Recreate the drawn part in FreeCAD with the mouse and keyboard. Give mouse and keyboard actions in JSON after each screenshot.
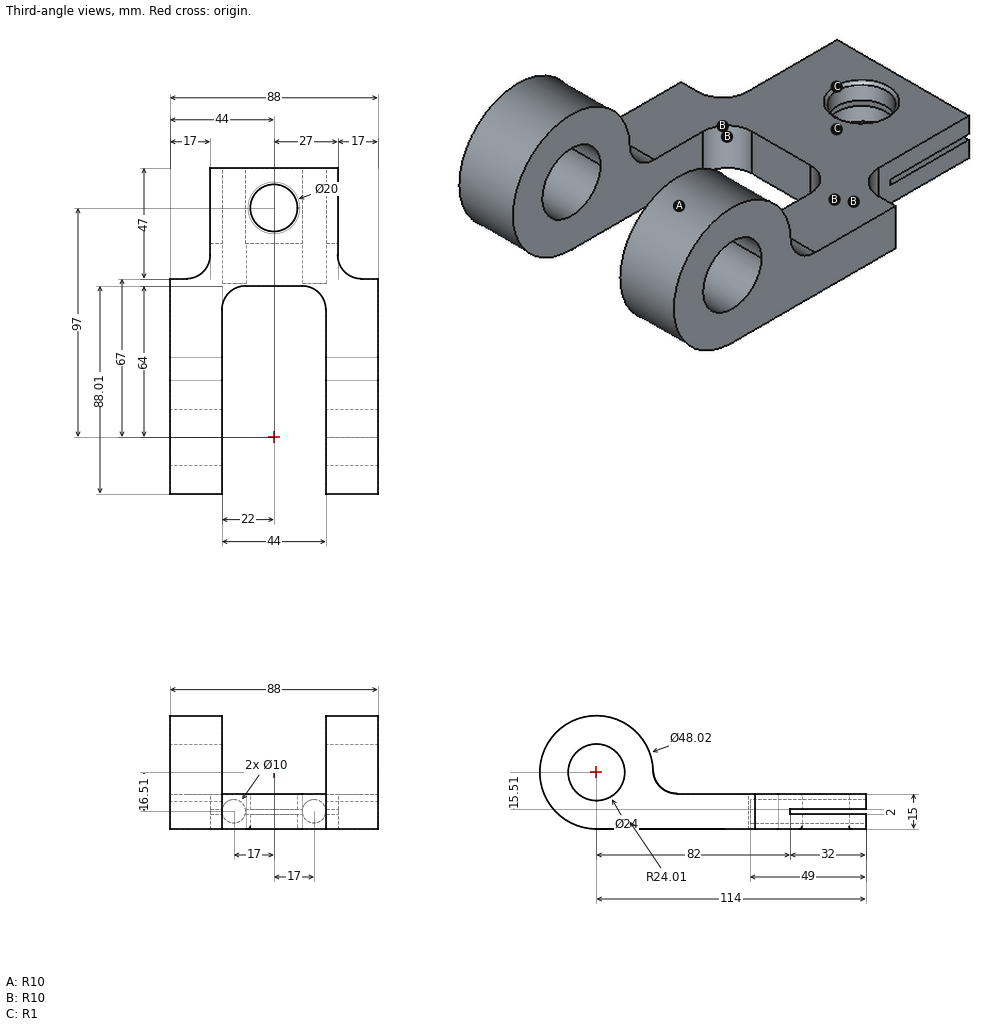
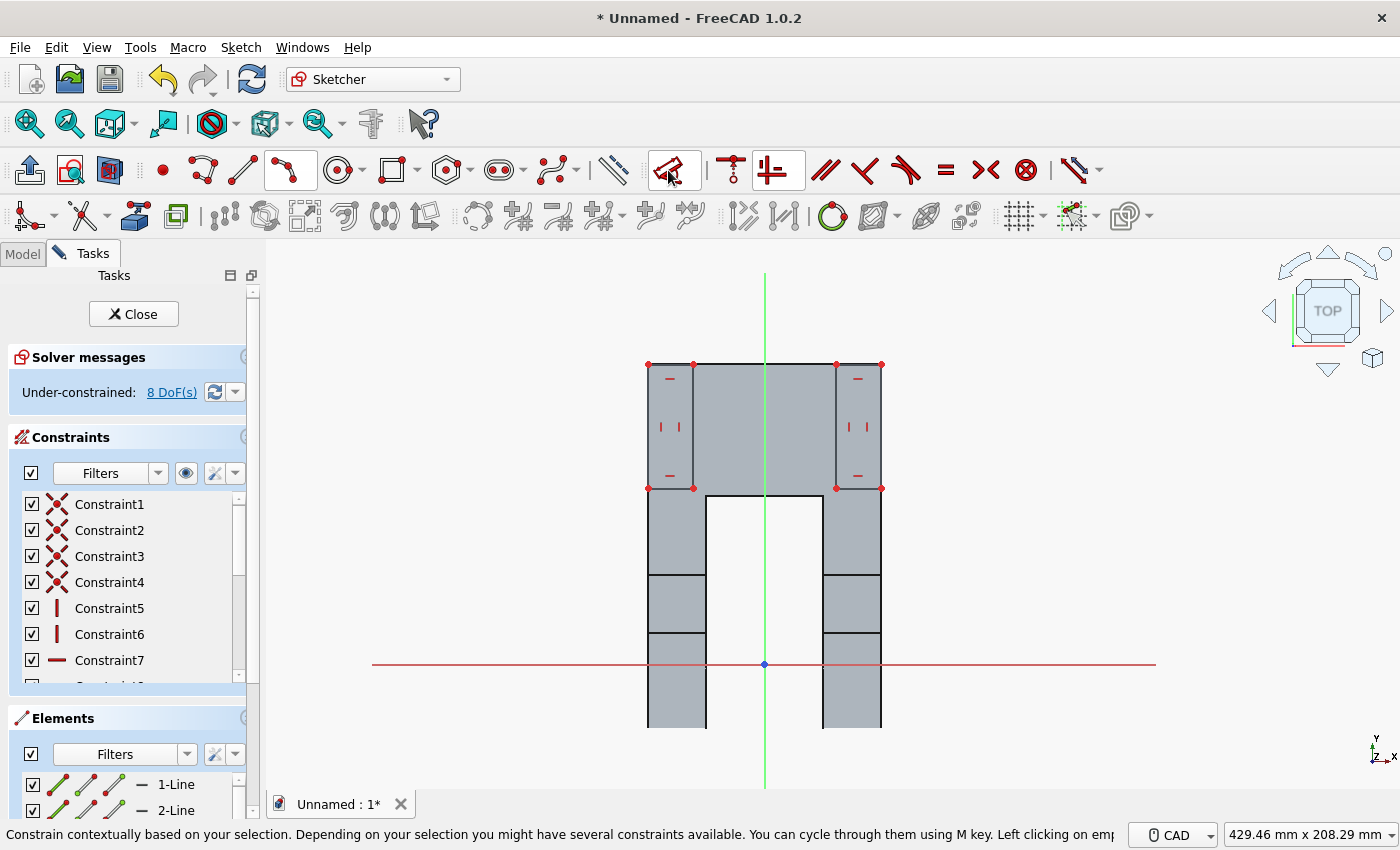
{"action": "left_click", "coordinate": [648, 402]}
{"action": "left_click", "coordinate": [614, 427]}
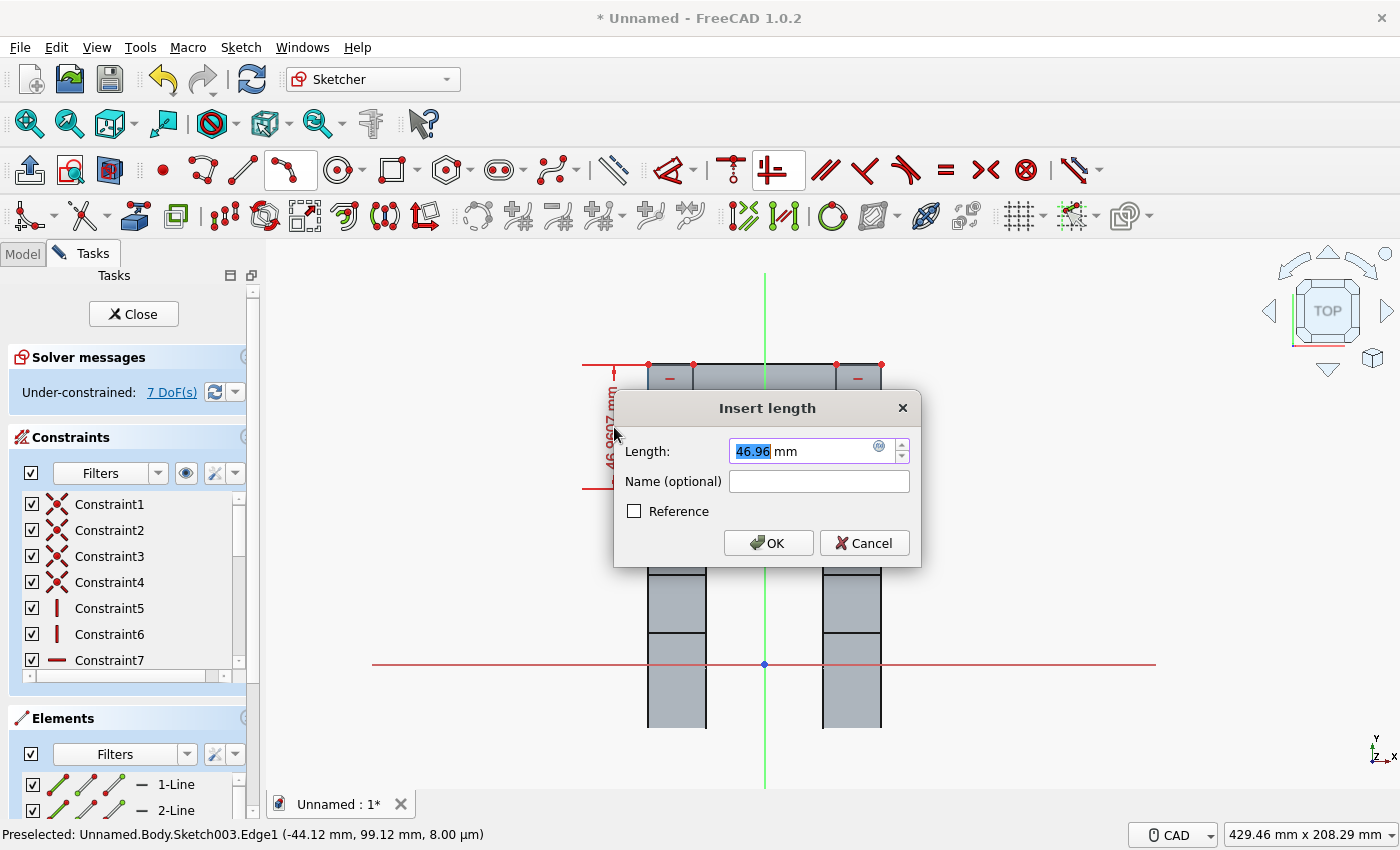
{"action": "type", "text": "47"}
{"action": "key", "text": "Return"}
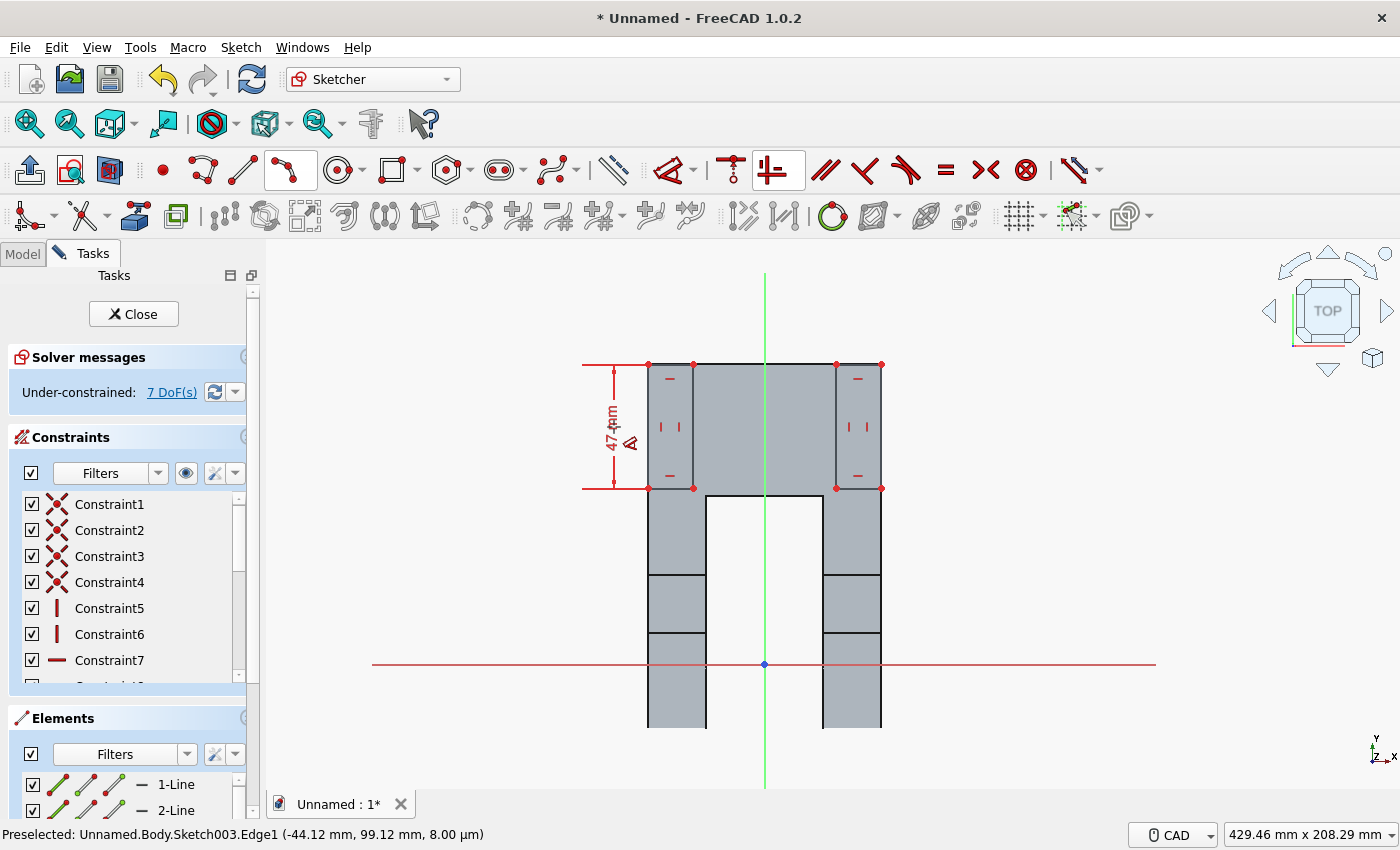
{"action": "left_click", "coordinate": [662, 489]}
{"action": "left_click", "coordinate": [671, 455]}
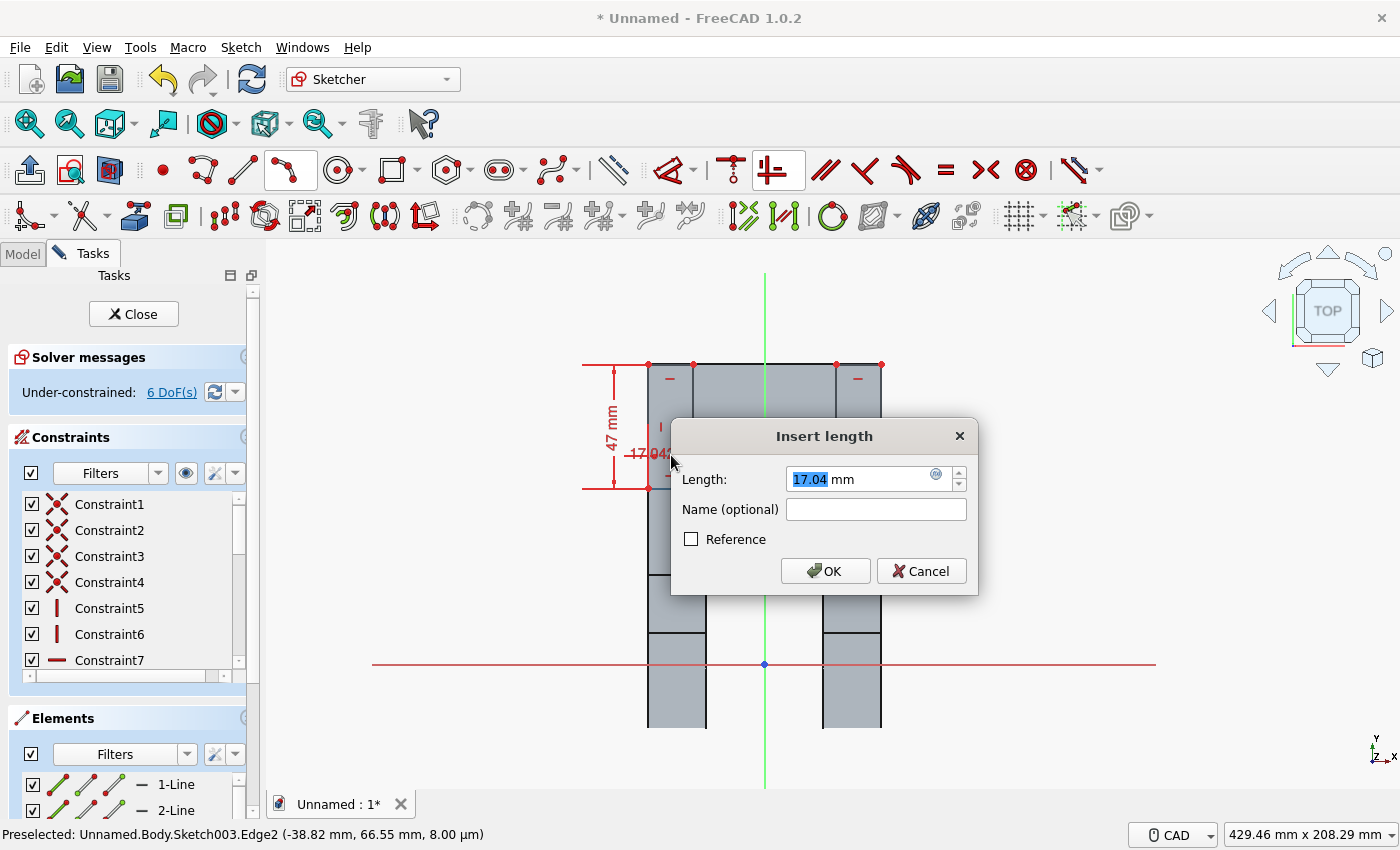
{"action": "type", "text": "17"}
{"action": "key", "text": "Return"}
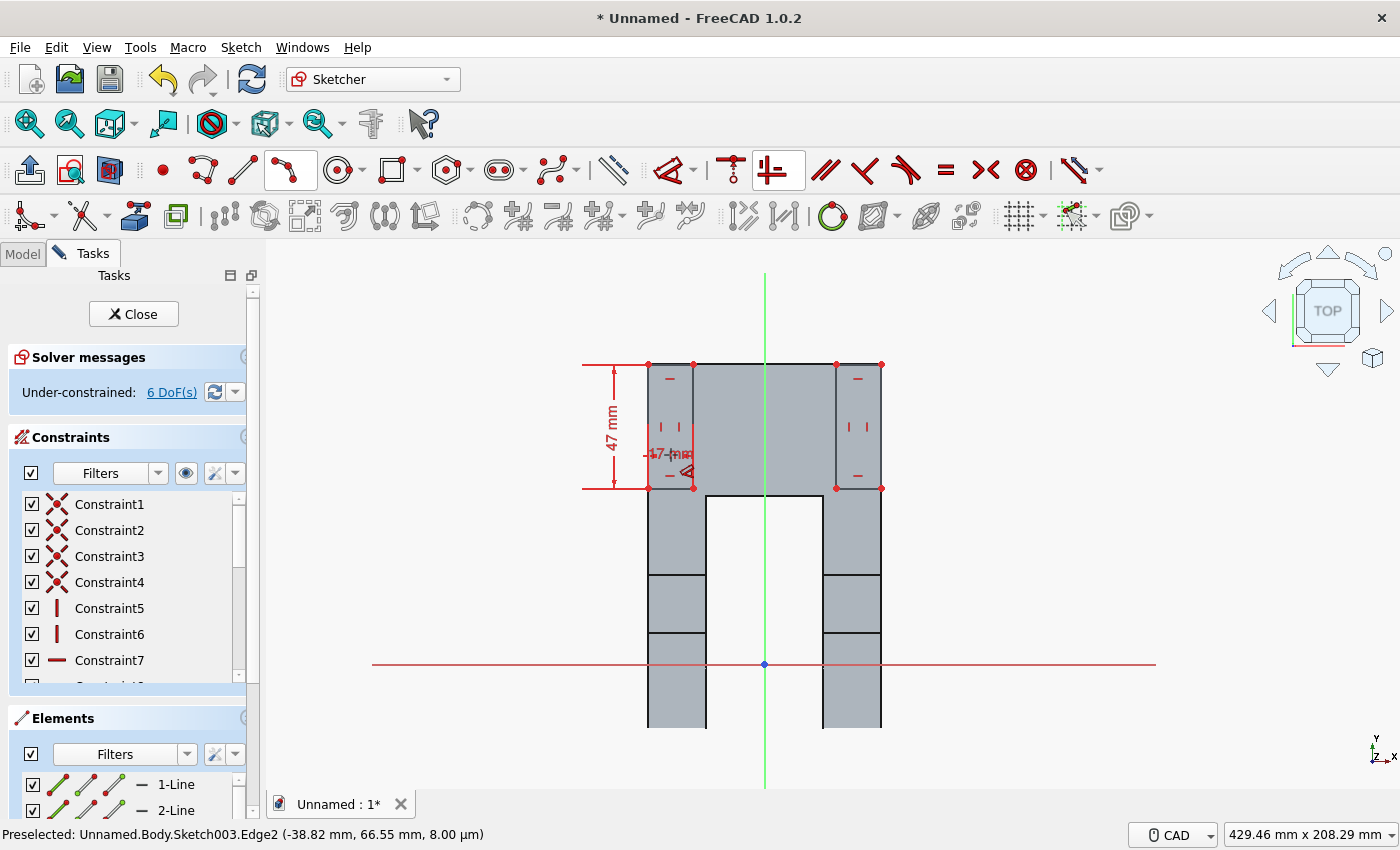
{"action": "left_click", "coordinate": [836, 402]}
{"action": "left_click", "coordinate": [802, 427]}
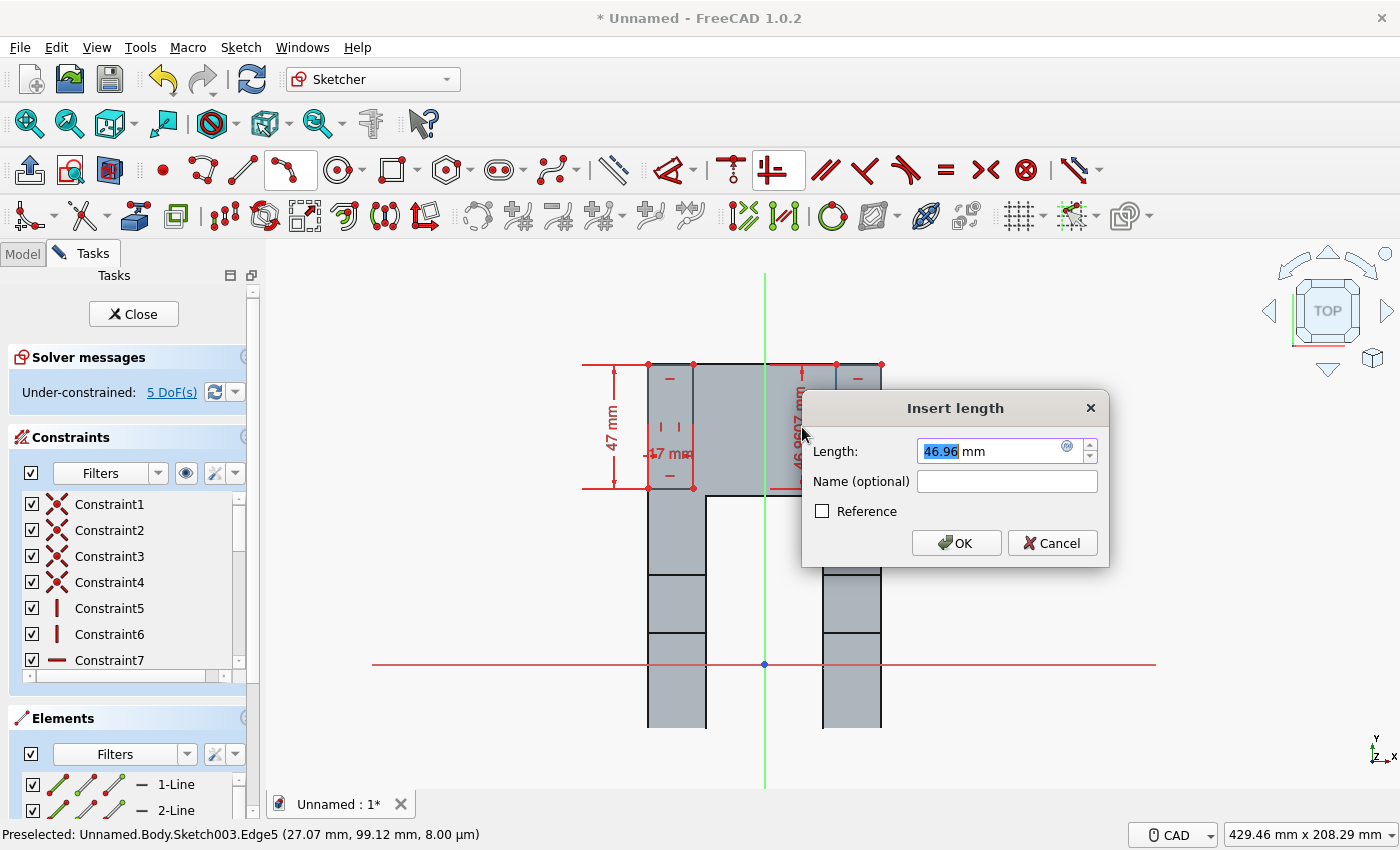
{"action": "type", "text": "47"}
{"action": "key", "text": "Return"}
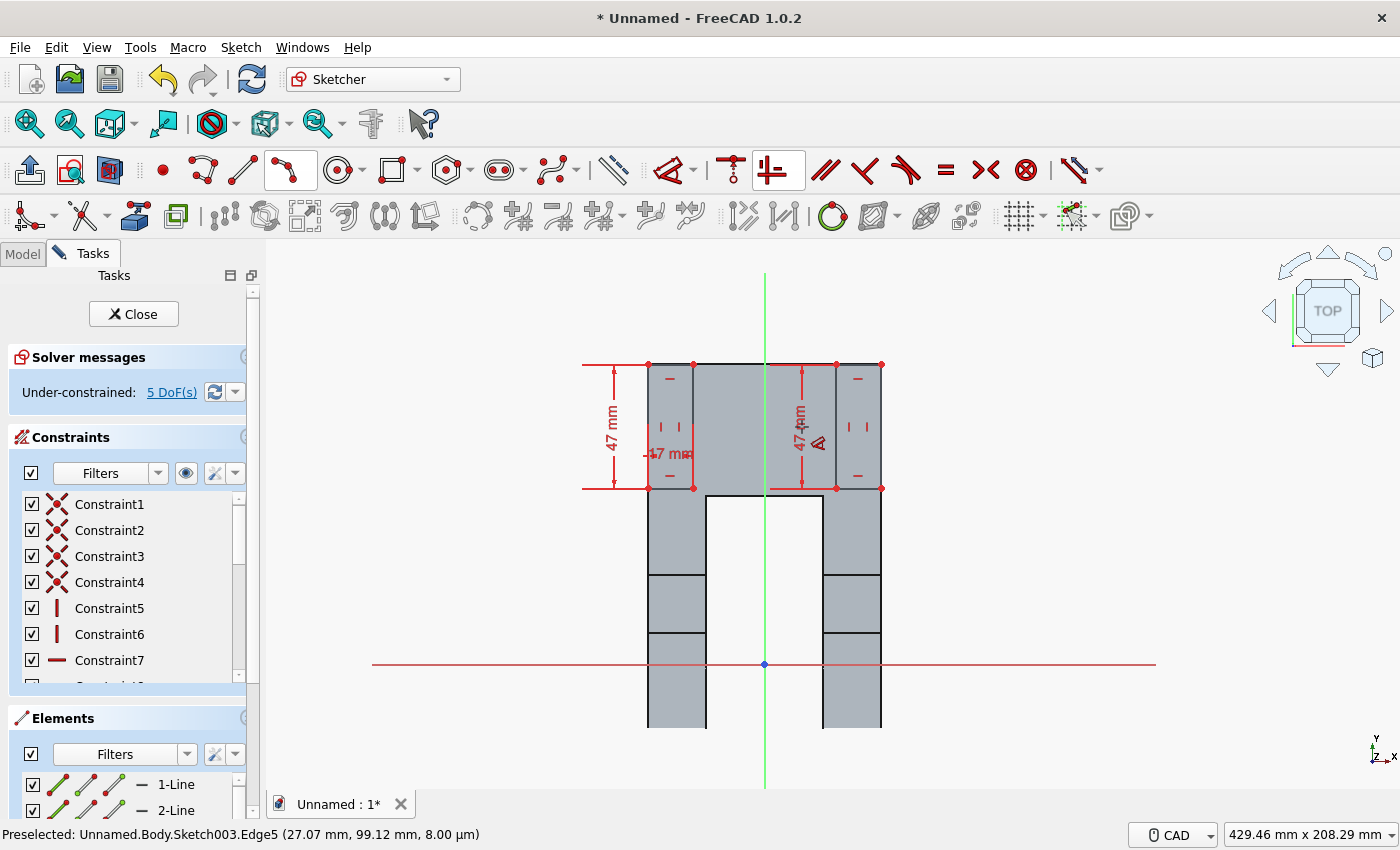
{"action": "left_click", "coordinate": [850, 489]}
{"action": "left_click", "coordinate": [859, 455]}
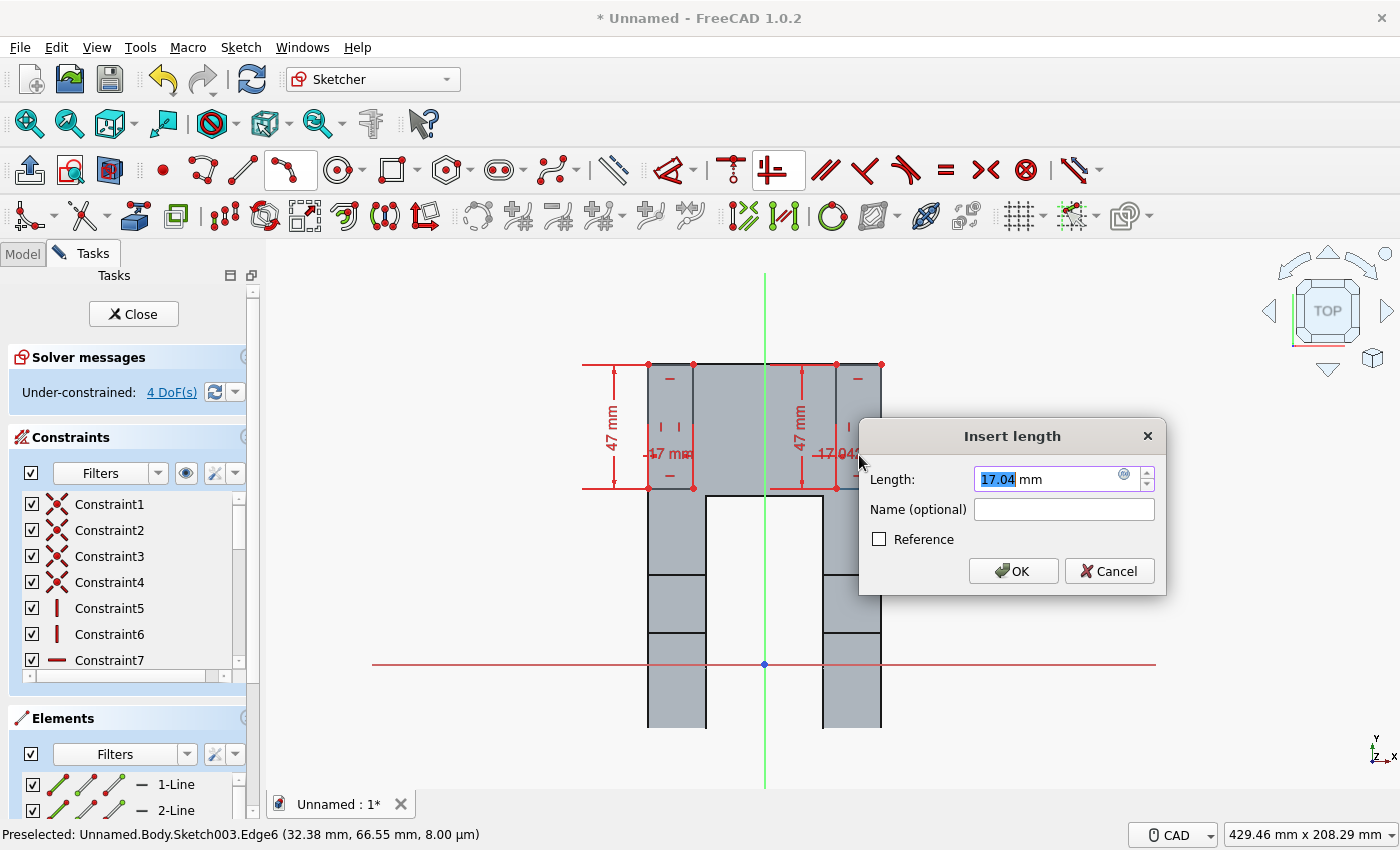
{"action": "type", "text": "17"}
{"action": "key", "text": "Return"}